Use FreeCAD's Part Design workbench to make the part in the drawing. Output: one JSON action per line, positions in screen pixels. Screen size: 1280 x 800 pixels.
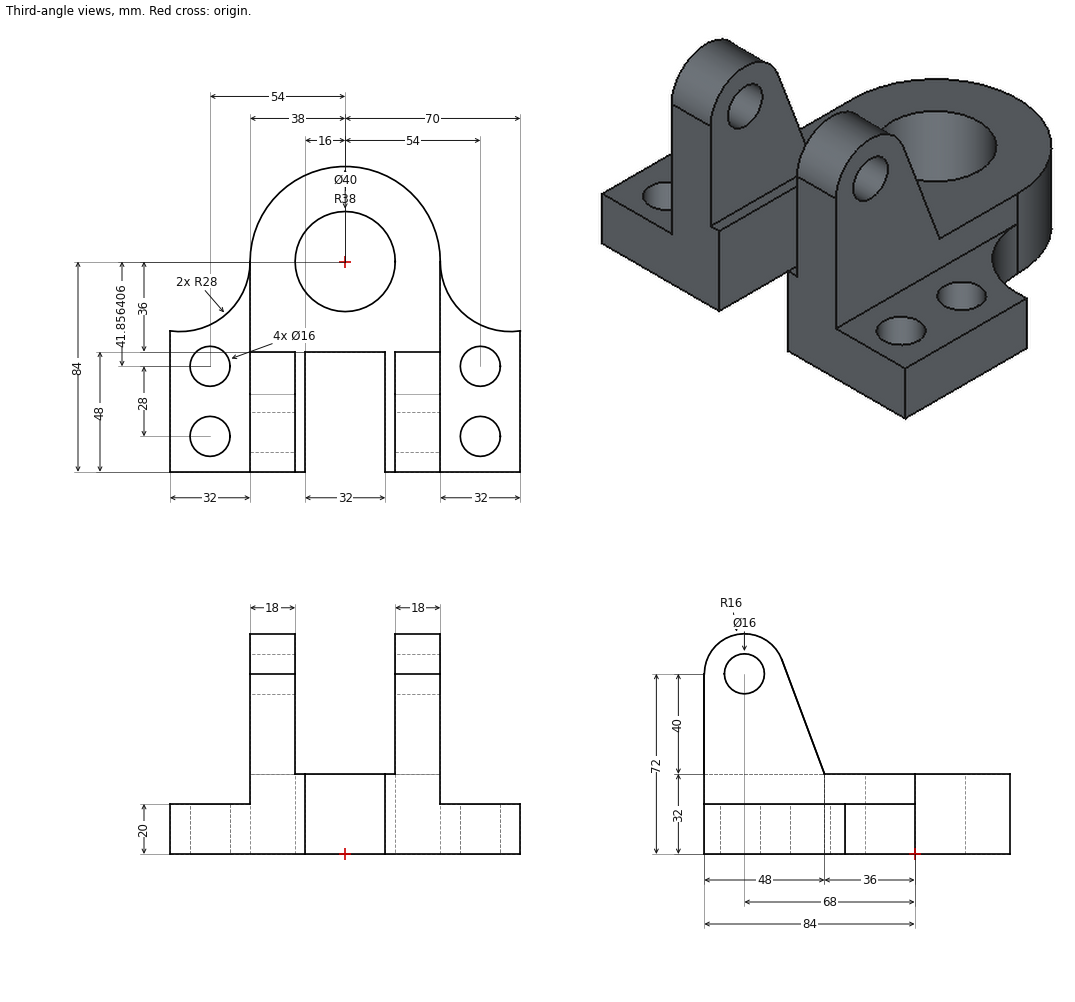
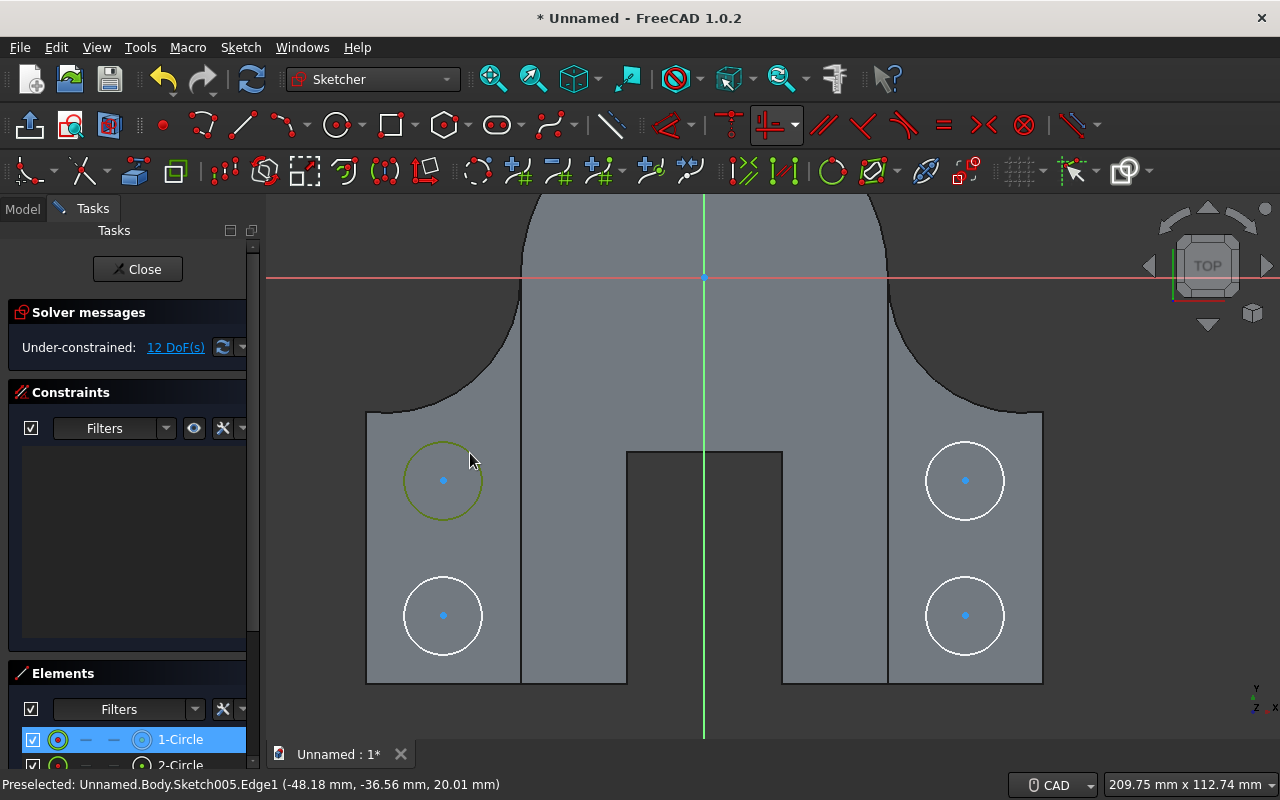
{"action": "left_click", "coordinate": [470, 588]}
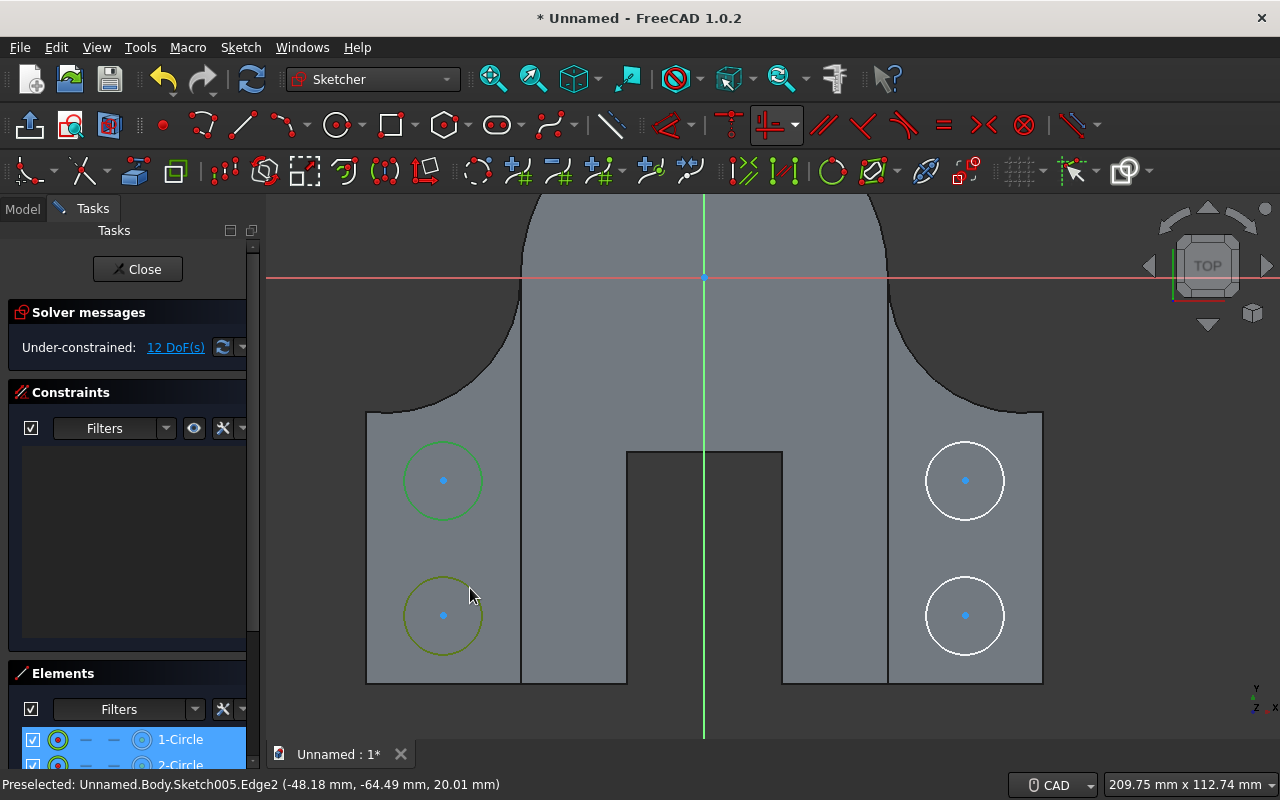
{"action": "left_click", "coordinate": [992, 453]}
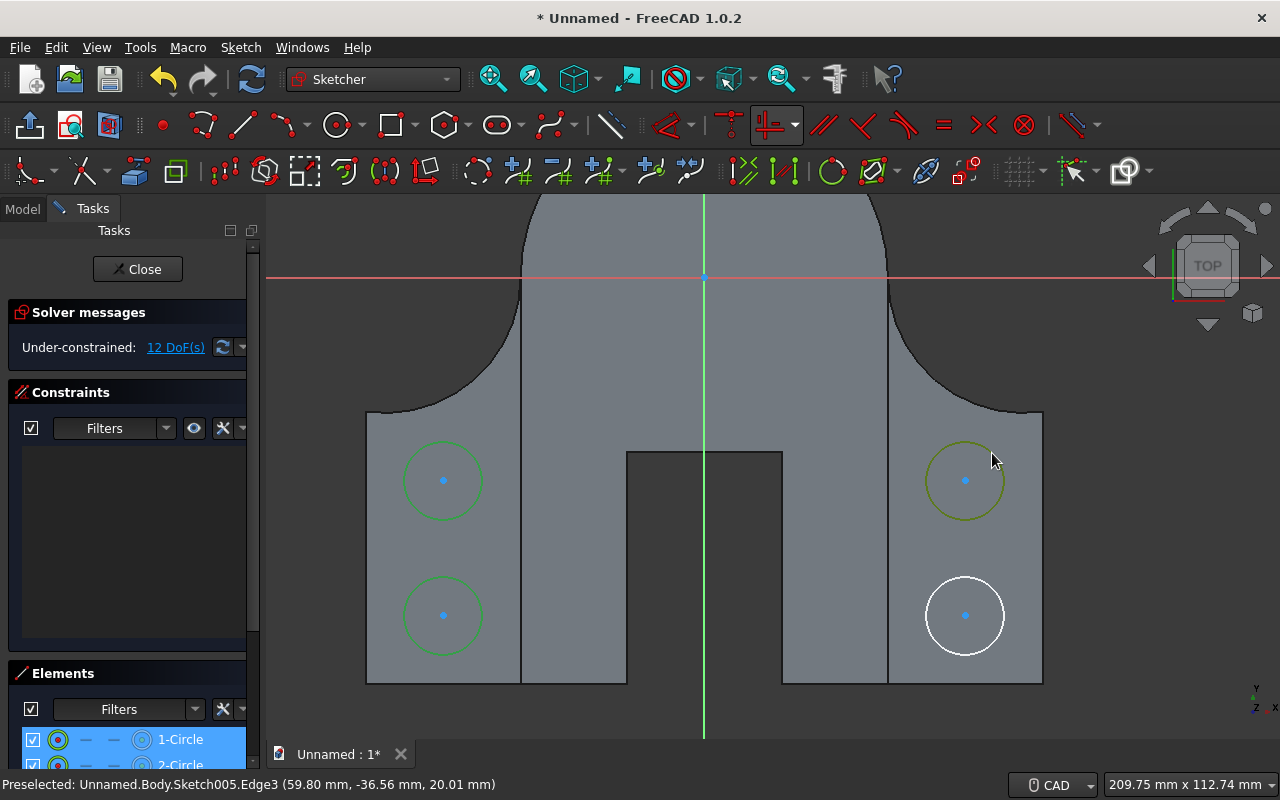
{"action": "left_click", "coordinate": [992, 588]}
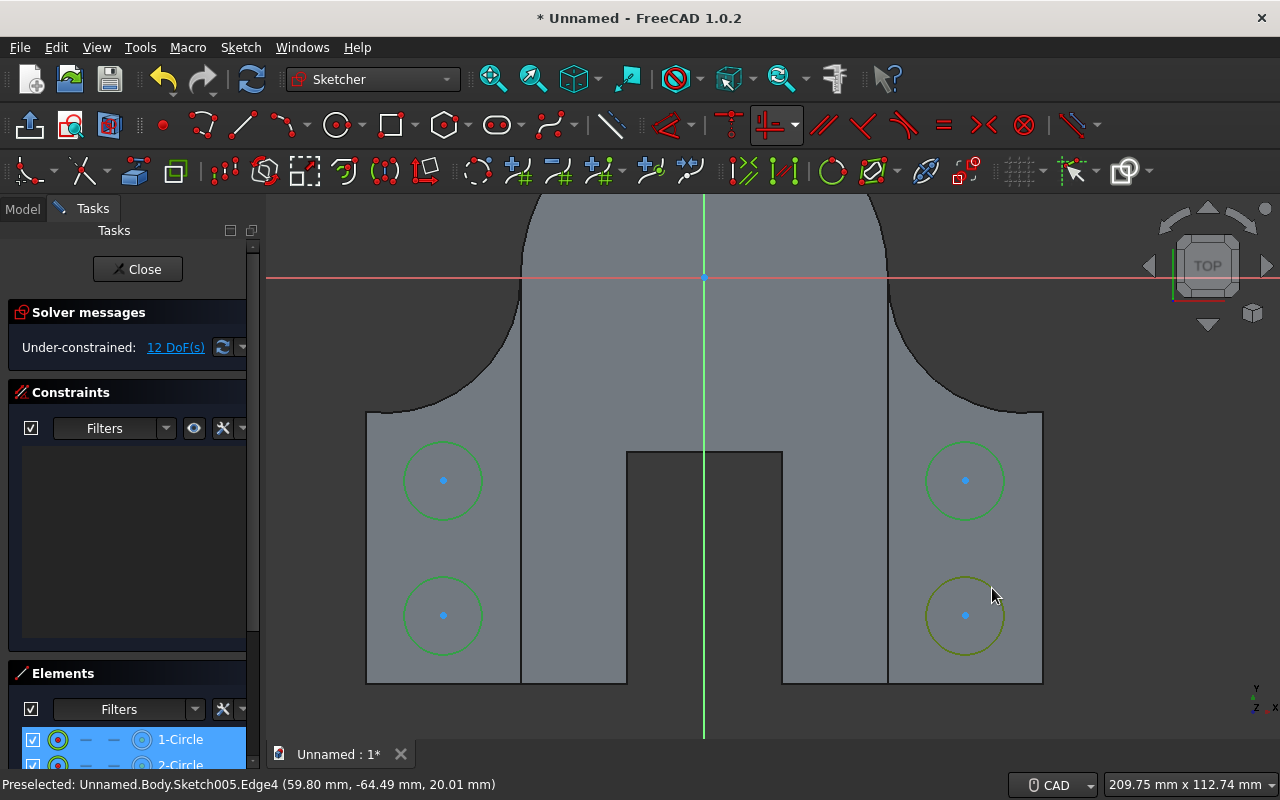
{"action": "left_click", "coordinate": [944, 126]}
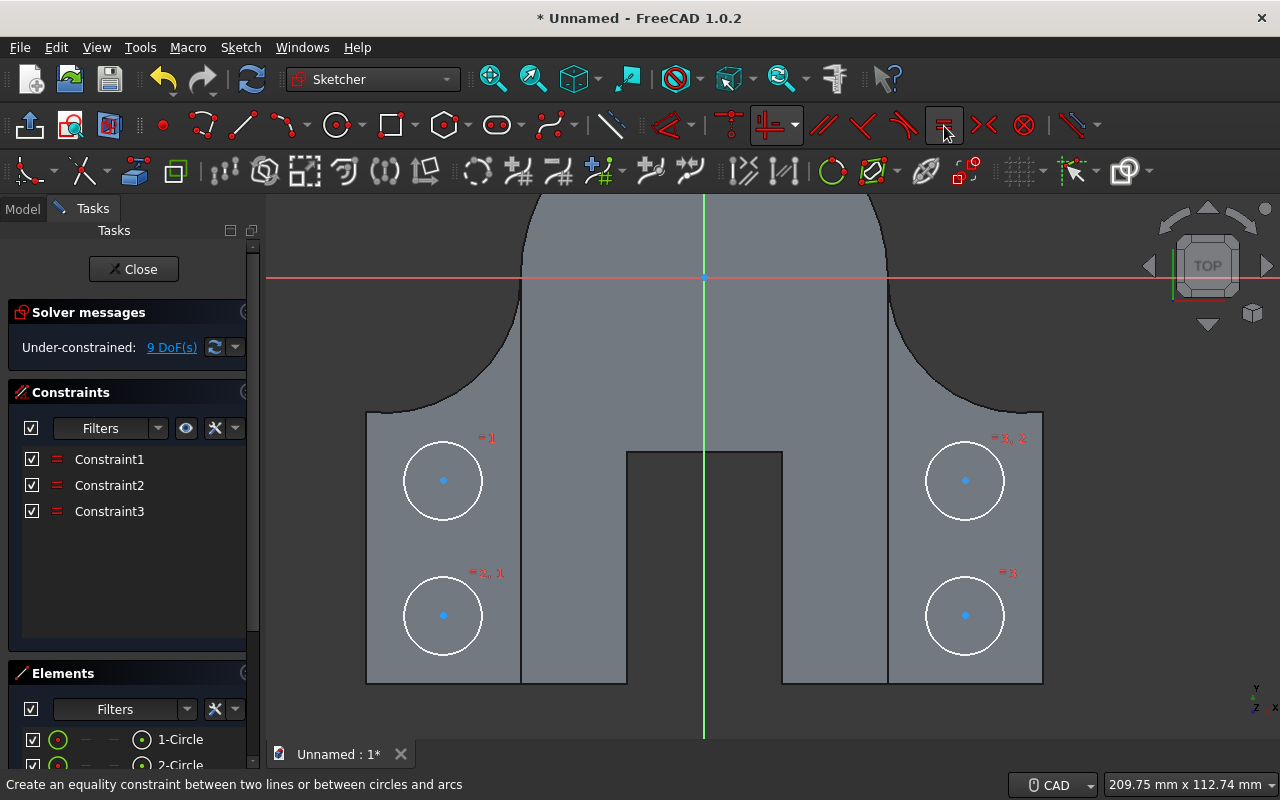
{"action": "left_click", "coordinate": [443, 481]}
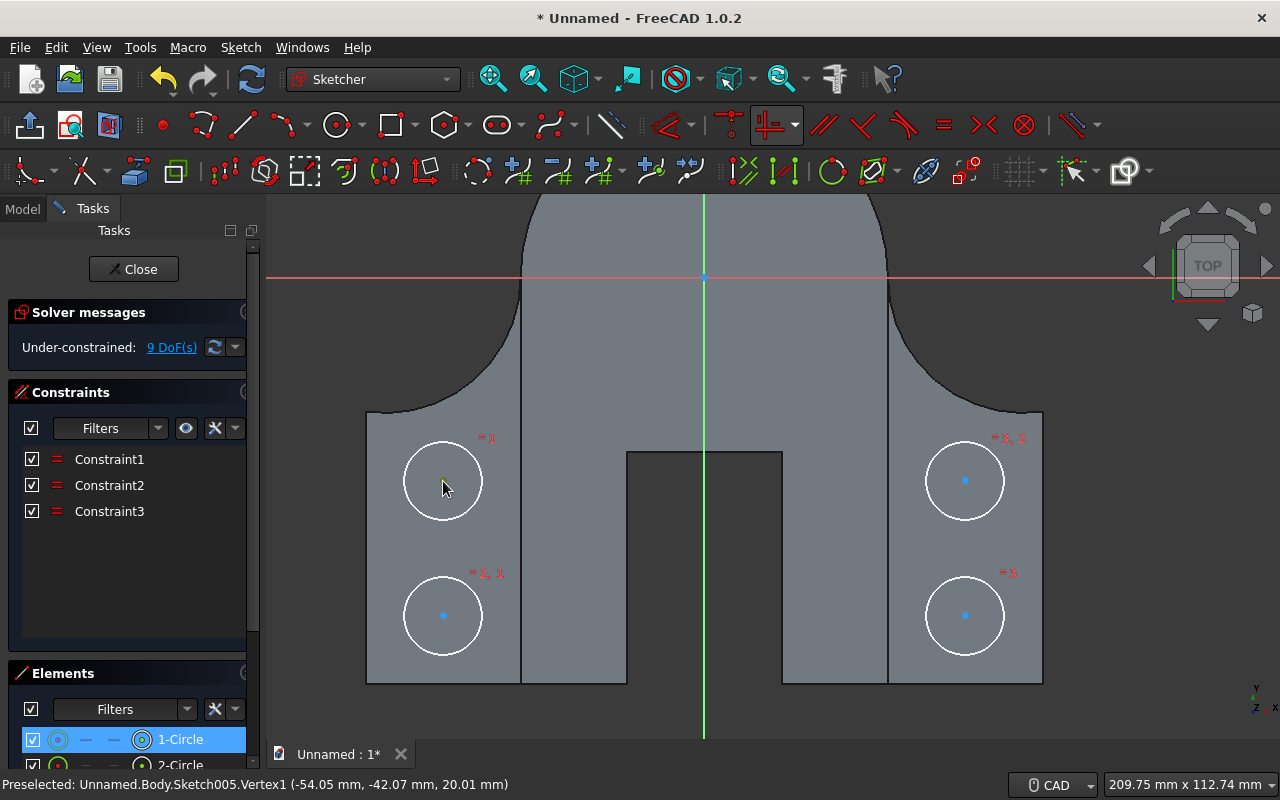
{"action": "left_click", "coordinate": [443, 616]}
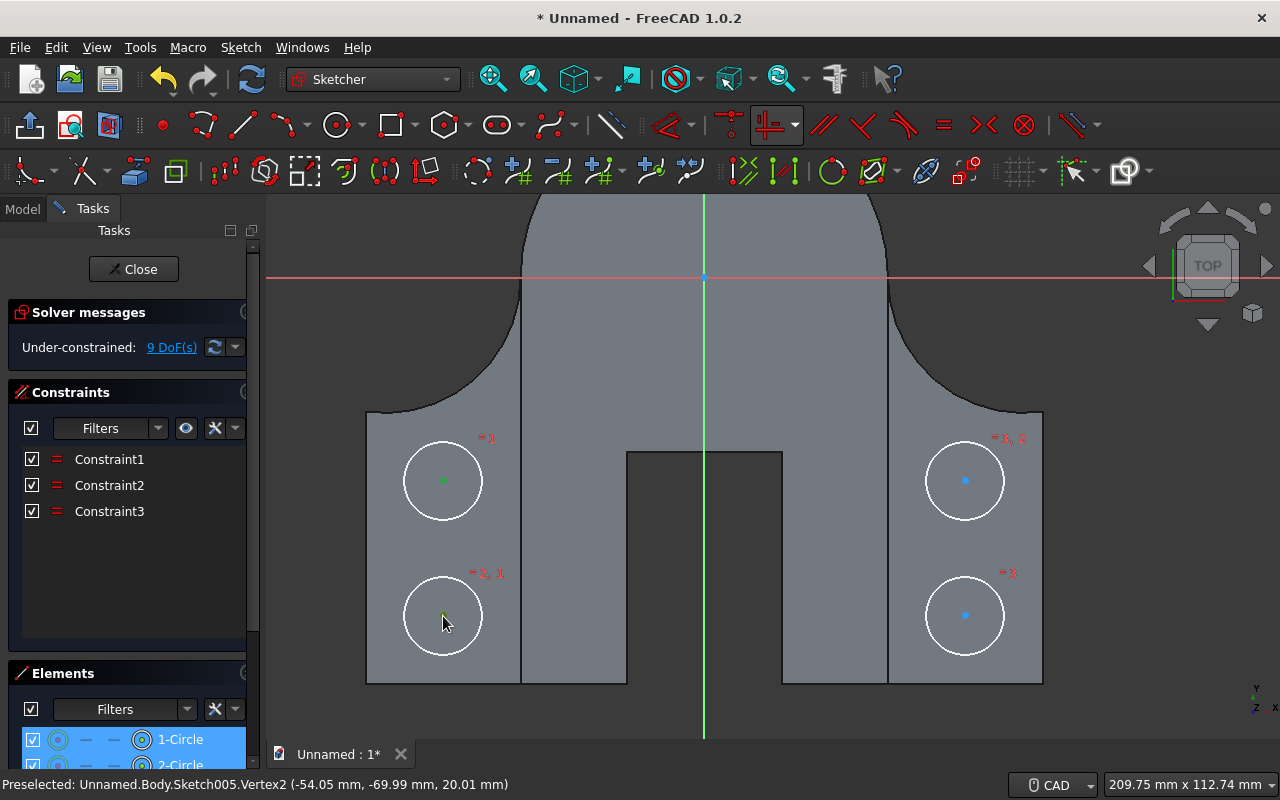
{"action": "key", "text": "v"}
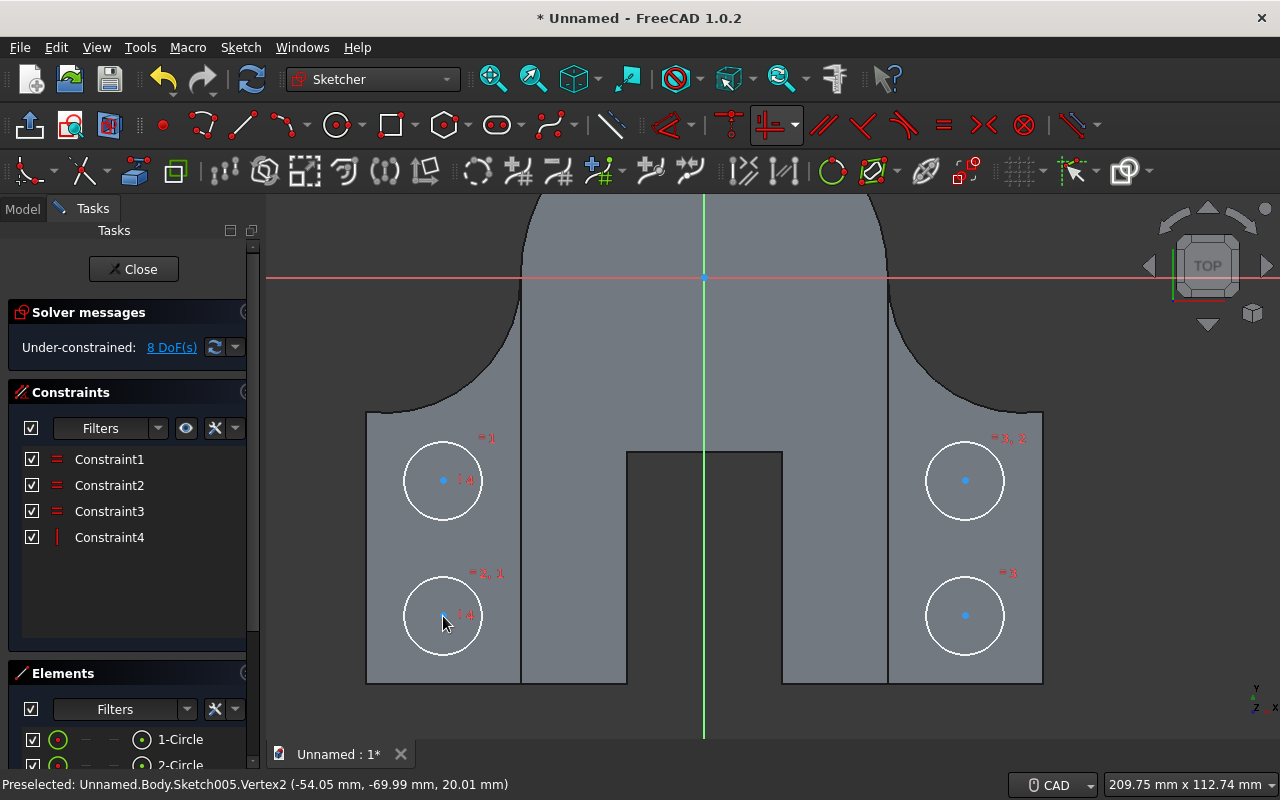
{"action": "left_click", "coordinate": [443, 481]}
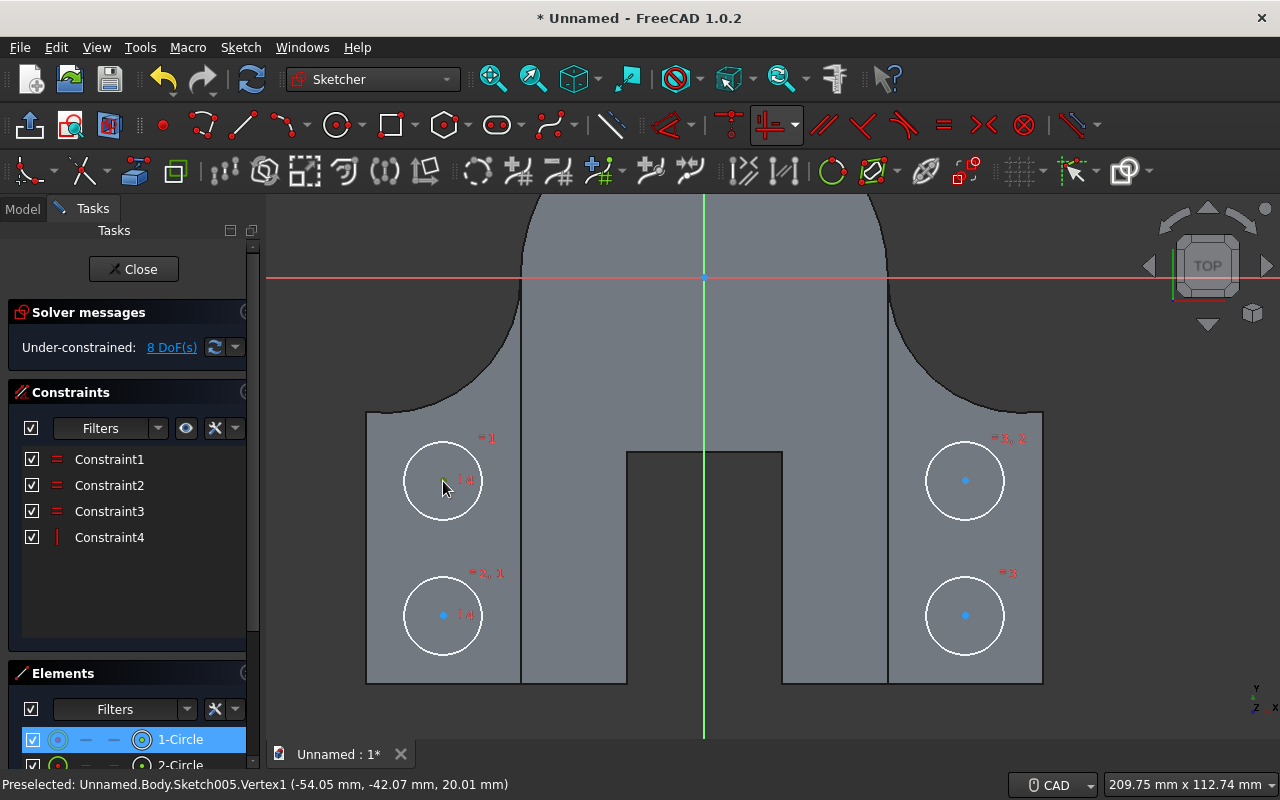
{"action": "left_click", "coordinate": [965, 481]}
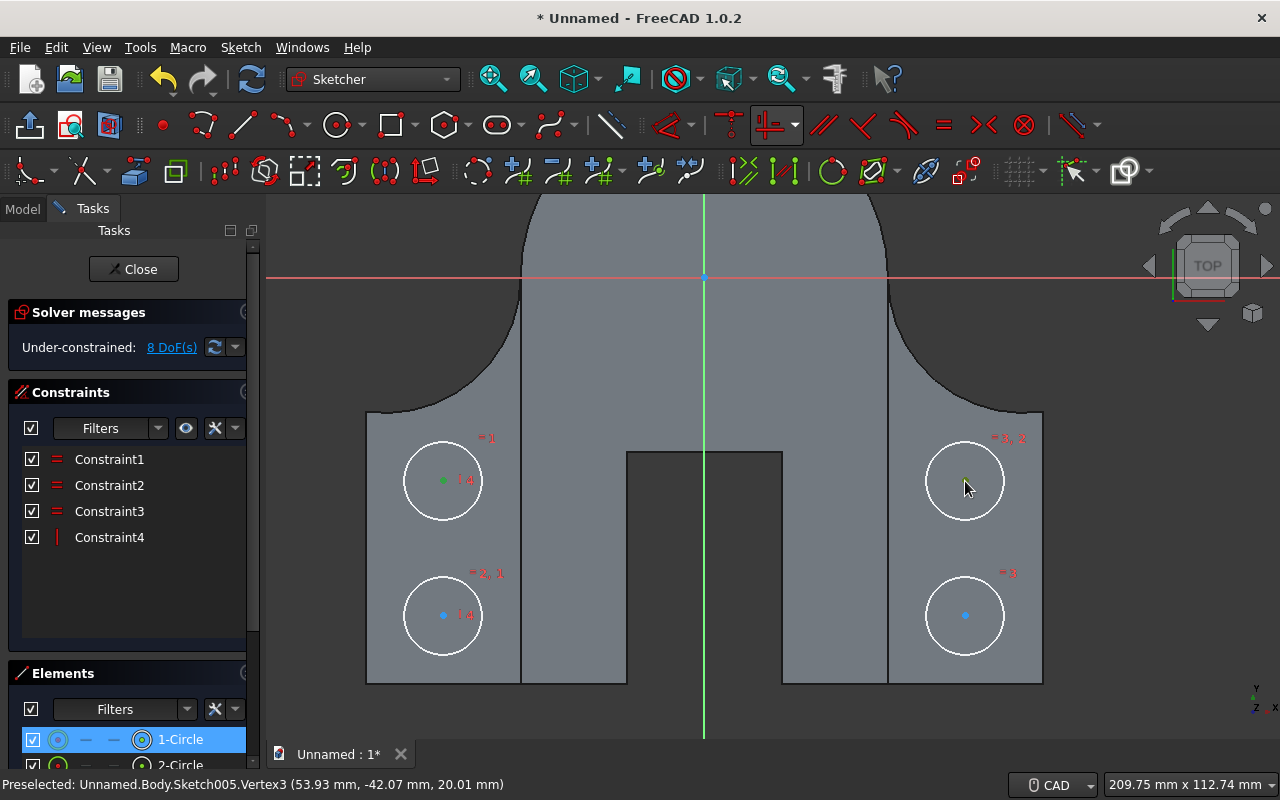
{"action": "left_click", "coordinate": [798, 126]}